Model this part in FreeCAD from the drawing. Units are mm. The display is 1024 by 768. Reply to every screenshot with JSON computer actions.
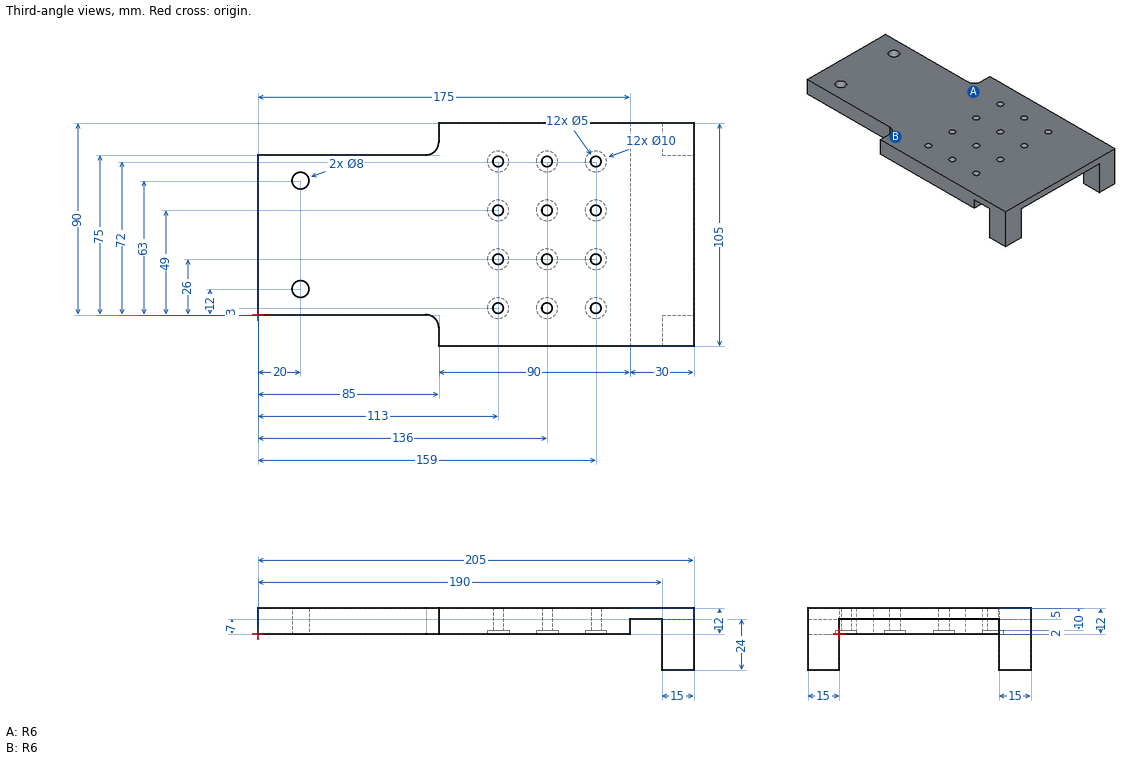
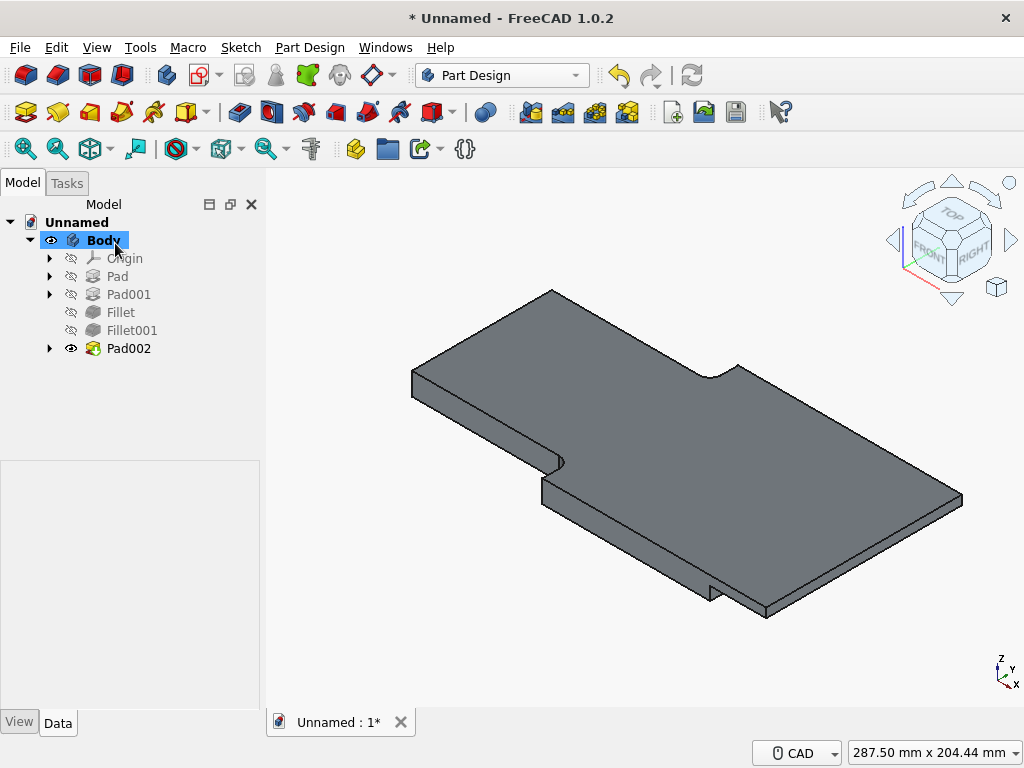
{"action": "key", "text": "4"}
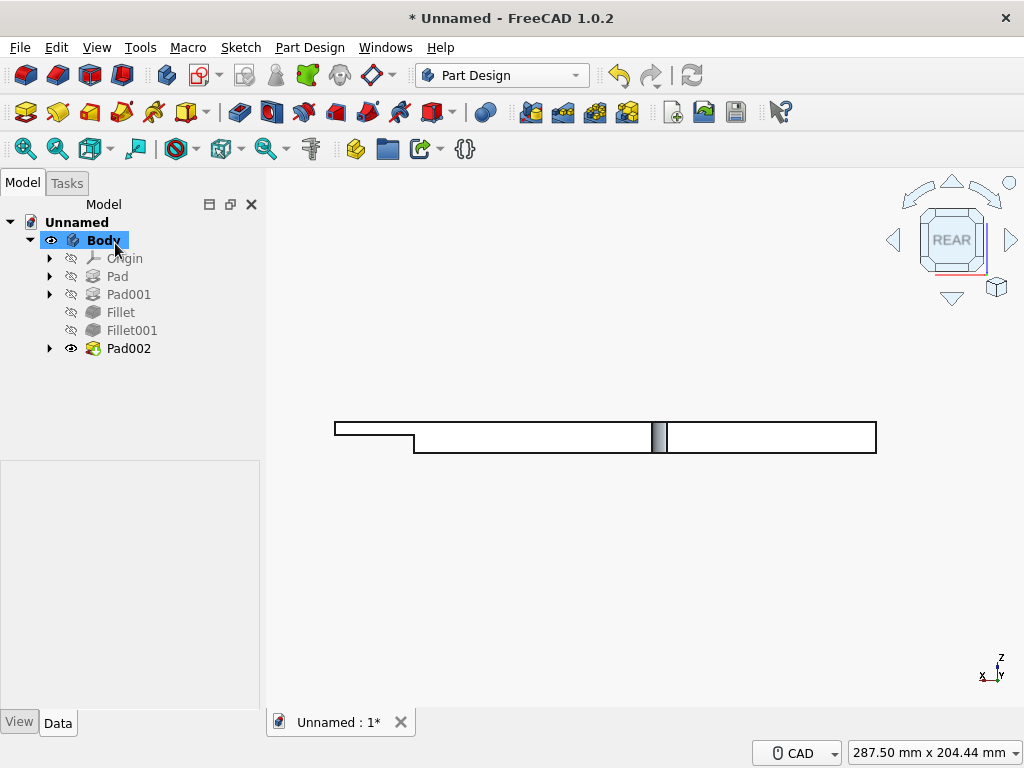
{"action": "left_click", "coordinate": [448, 437]}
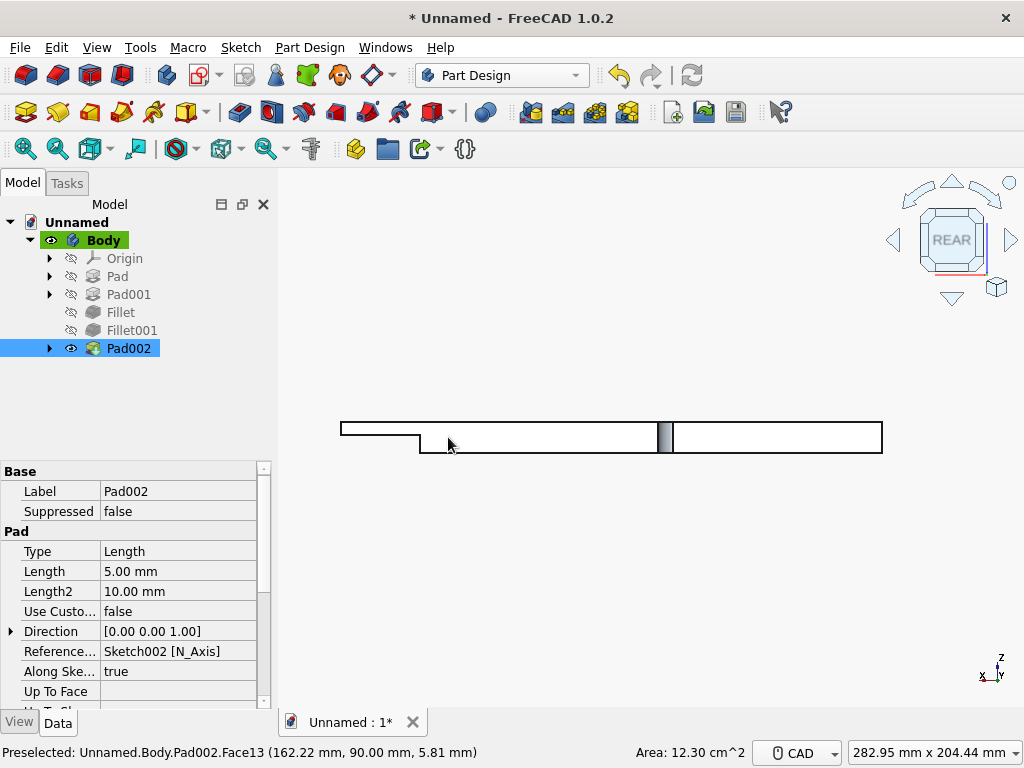
{"action": "left_click", "coordinate": [200, 76]}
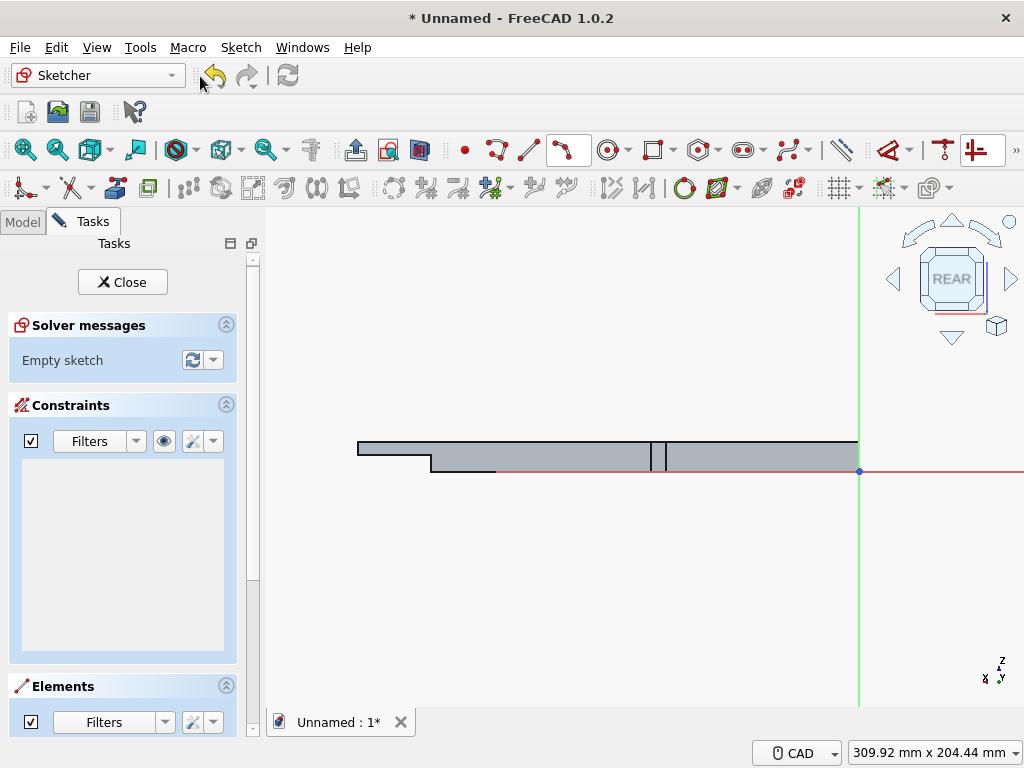
{"action": "scroll", "coordinate": [325, 491], "scroll_direction": "up", "scroll_amount": 8}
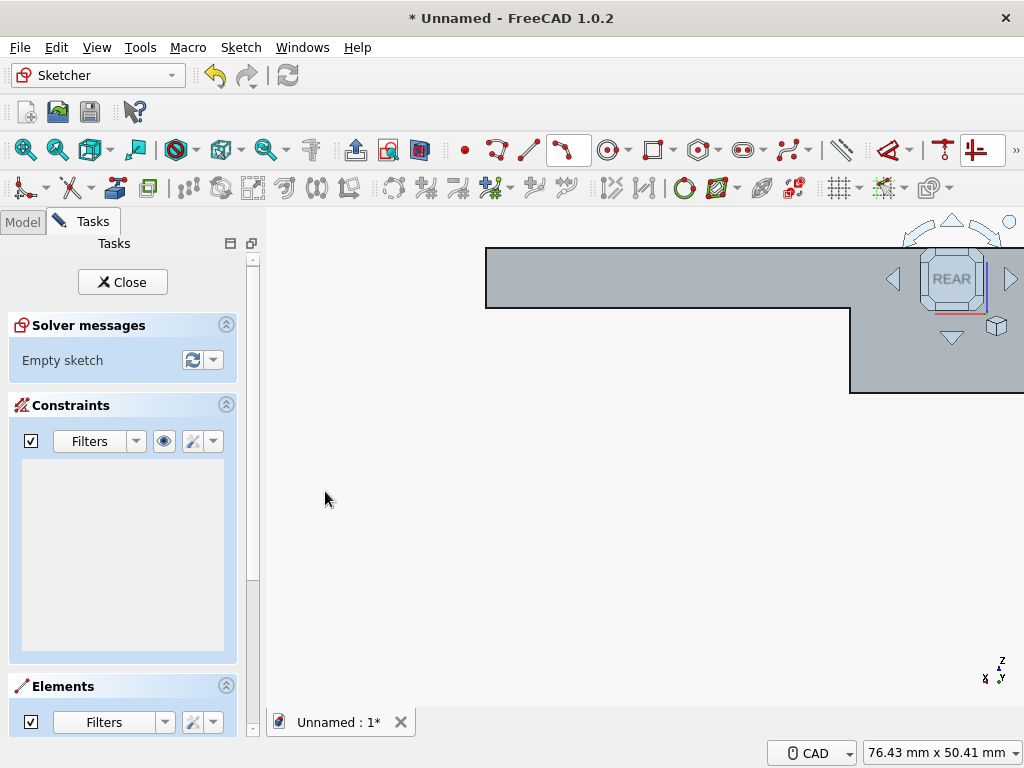
{"action": "left_click", "coordinate": [654, 150]}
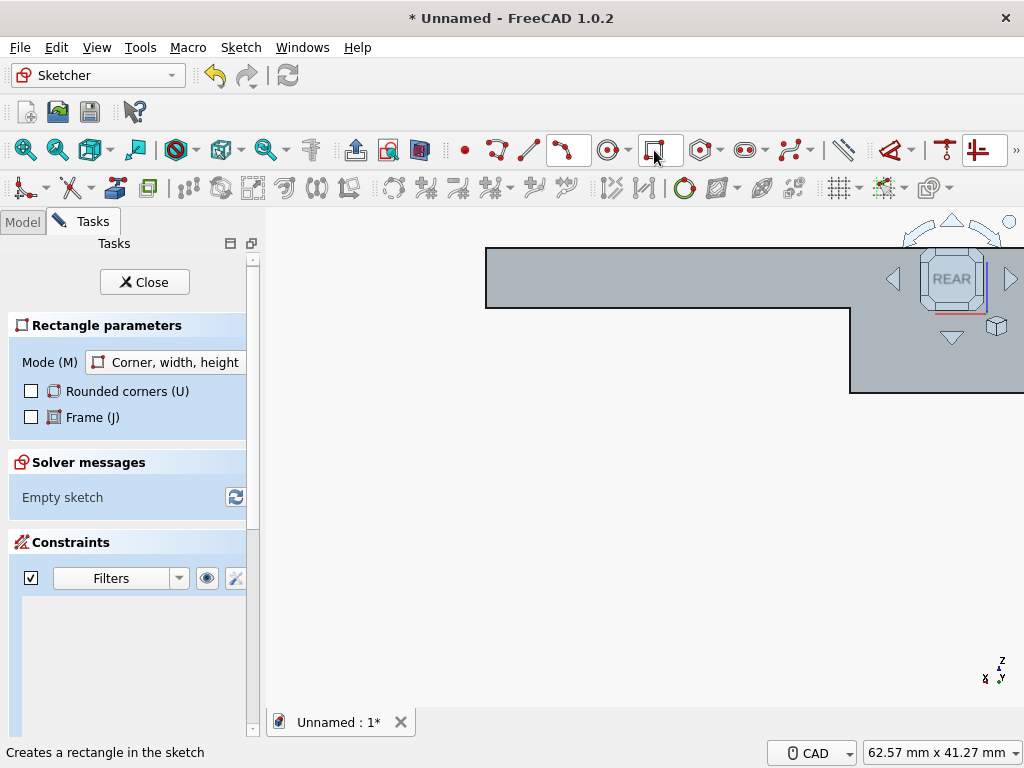
{"action": "left_click", "coordinate": [486, 308]}
{"action": "mouse_move", "coordinate": [668, 599]}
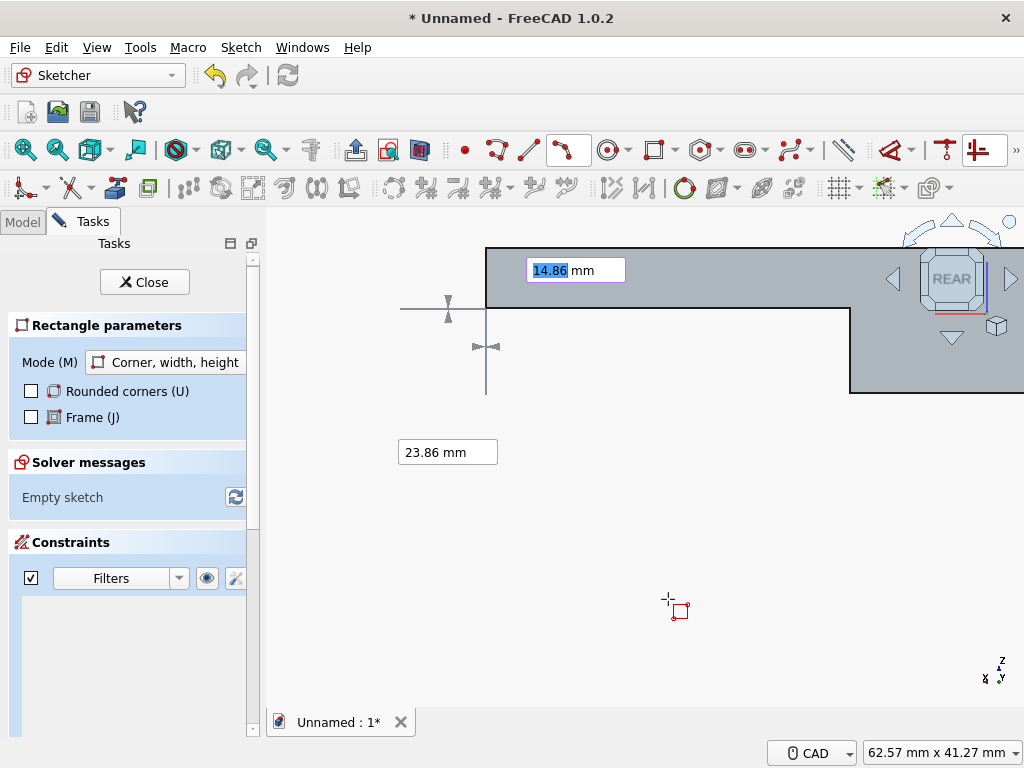
{"action": "type", "text": "15"}
{"action": "key", "text": "Tab"}
{"action": "type", "text": "24"}
{"action": "key", "text": "Return"}
{"action": "key", "text": "Escape"}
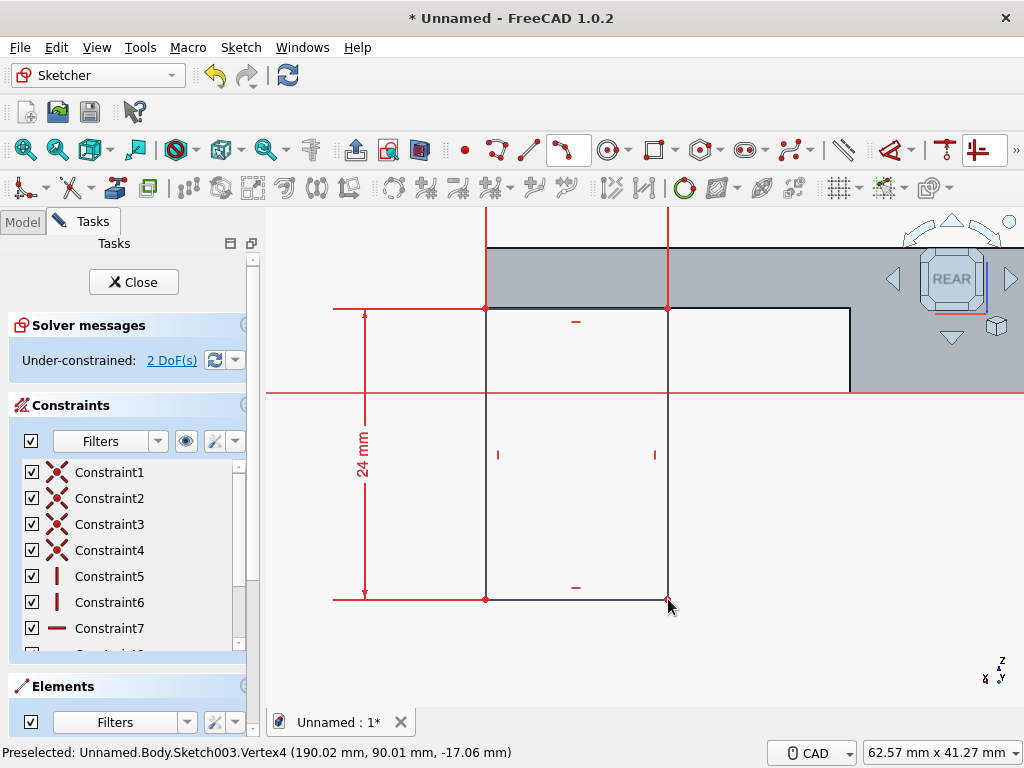
{"action": "left_click", "coordinate": [890, 150]}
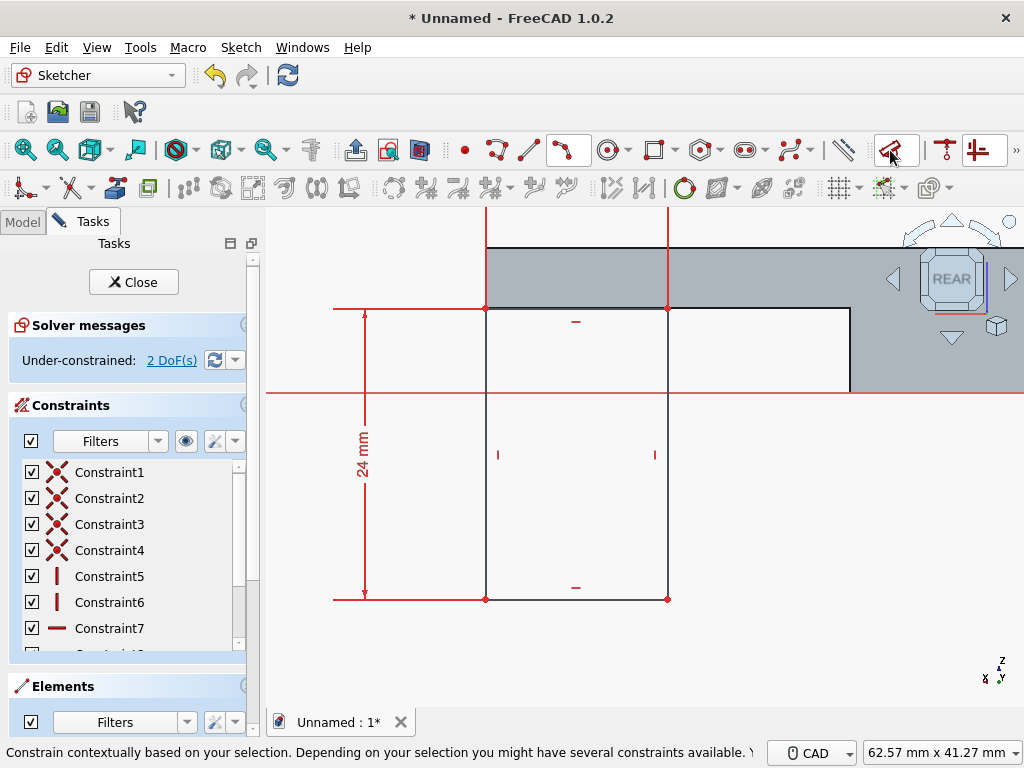
{"action": "left_click", "coordinate": [486, 309]}
{"action": "left_click", "coordinate": [452, 351]}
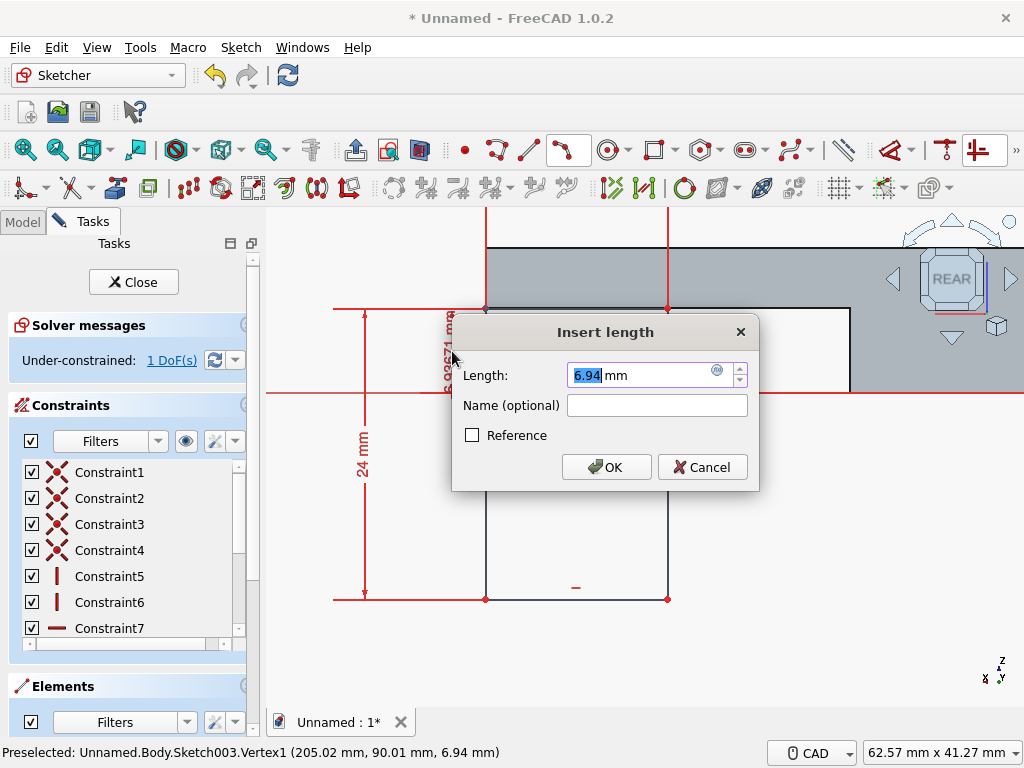
{"action": "type", "text": "7"}
{"action": "key", "text": "Return"}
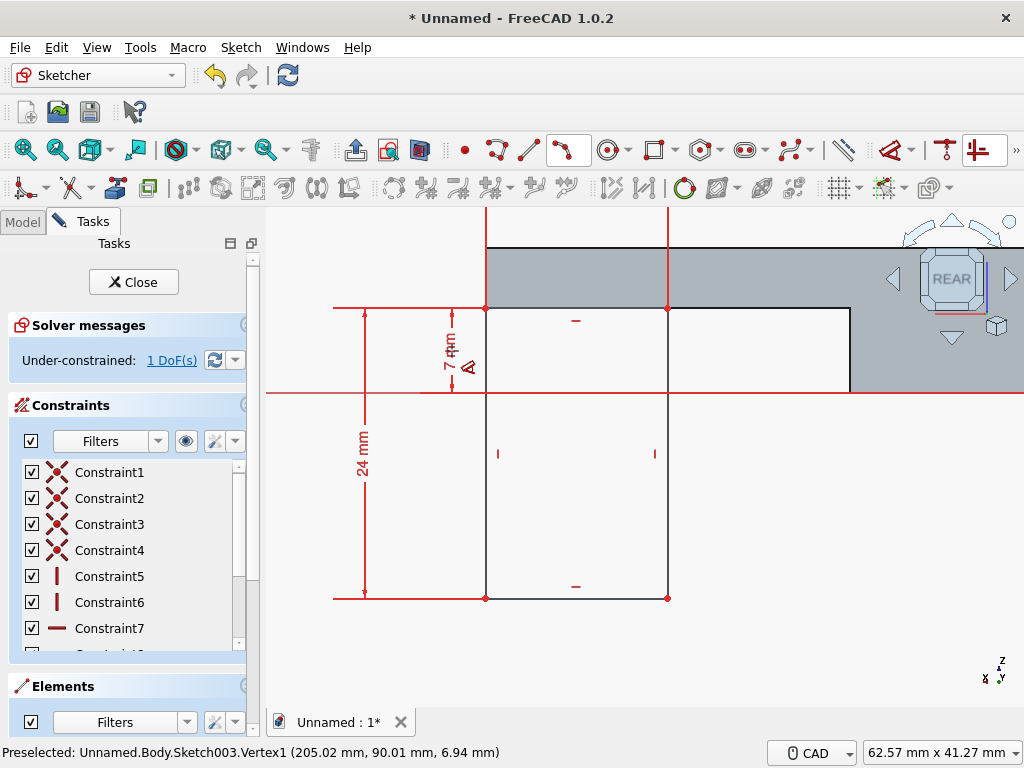
{"action": "left_click", "coordinate": [486, 308]}
{"action": "left_click", "coordinate": [673, 274]}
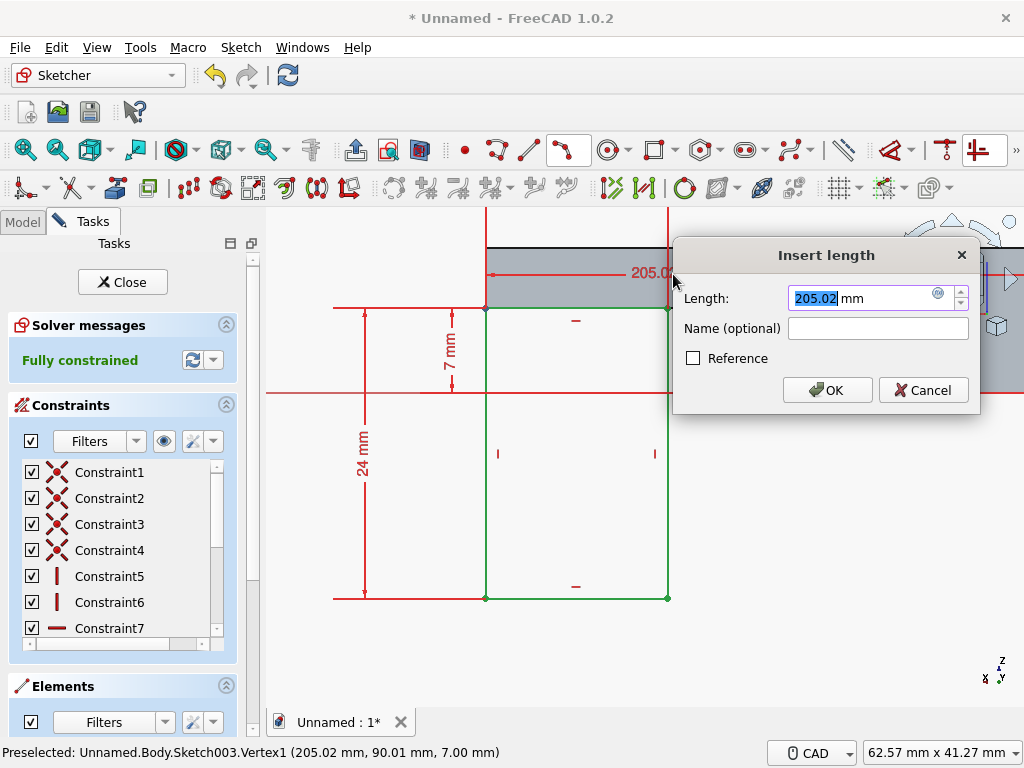
{"action": "type", "text": "205"}
{"action": "key", "text": "Return"}
{"action": "key", "text": "Escape"}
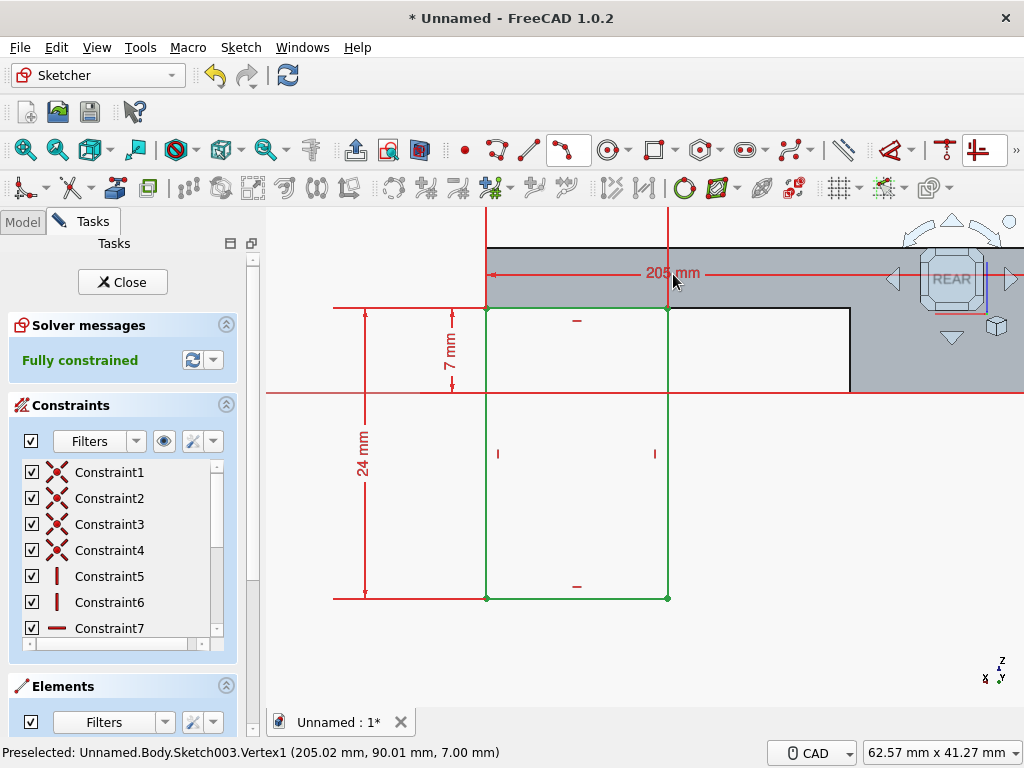
{"action": "left_click", "coordinate": [123, 282]}